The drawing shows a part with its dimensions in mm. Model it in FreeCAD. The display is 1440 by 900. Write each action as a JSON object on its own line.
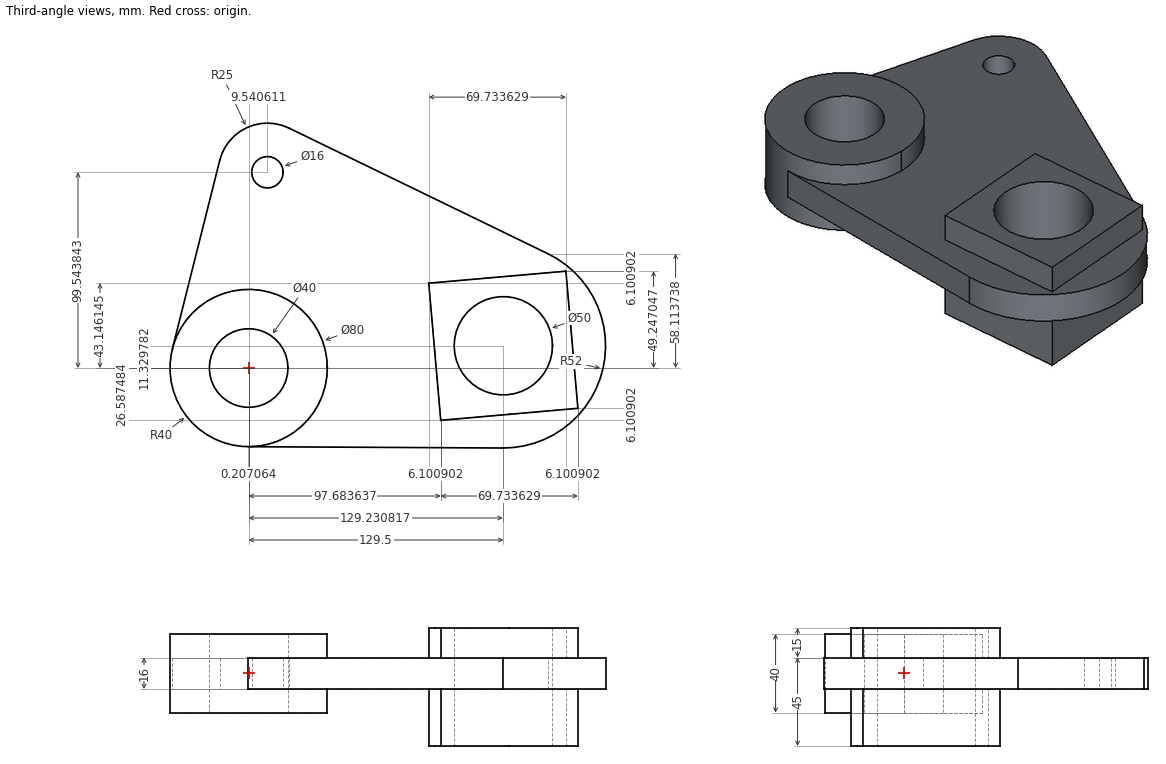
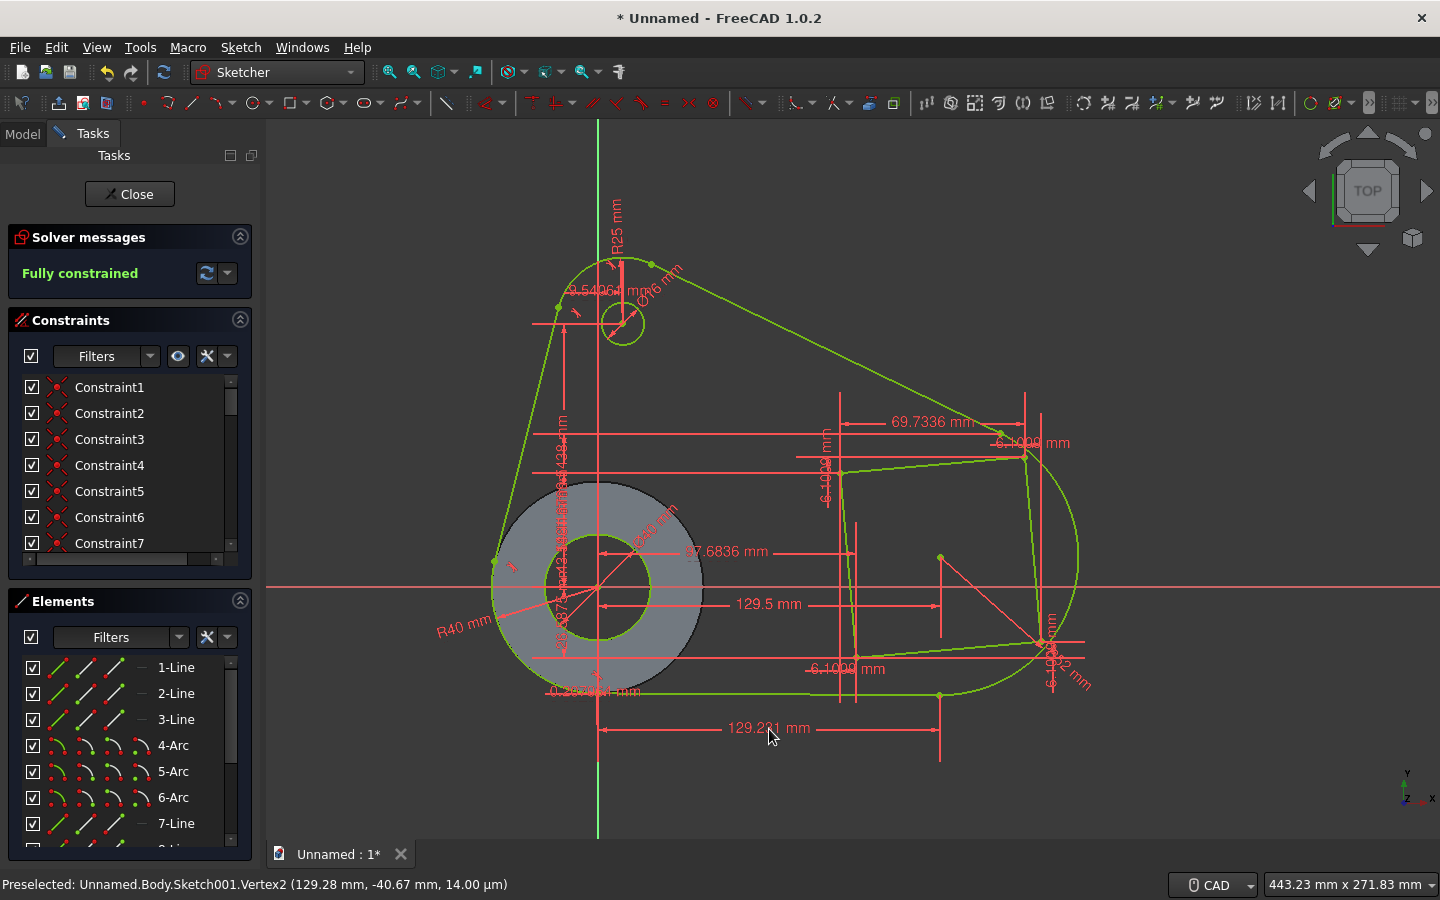
{"action": "left_click", "coordinate": [130, 194]}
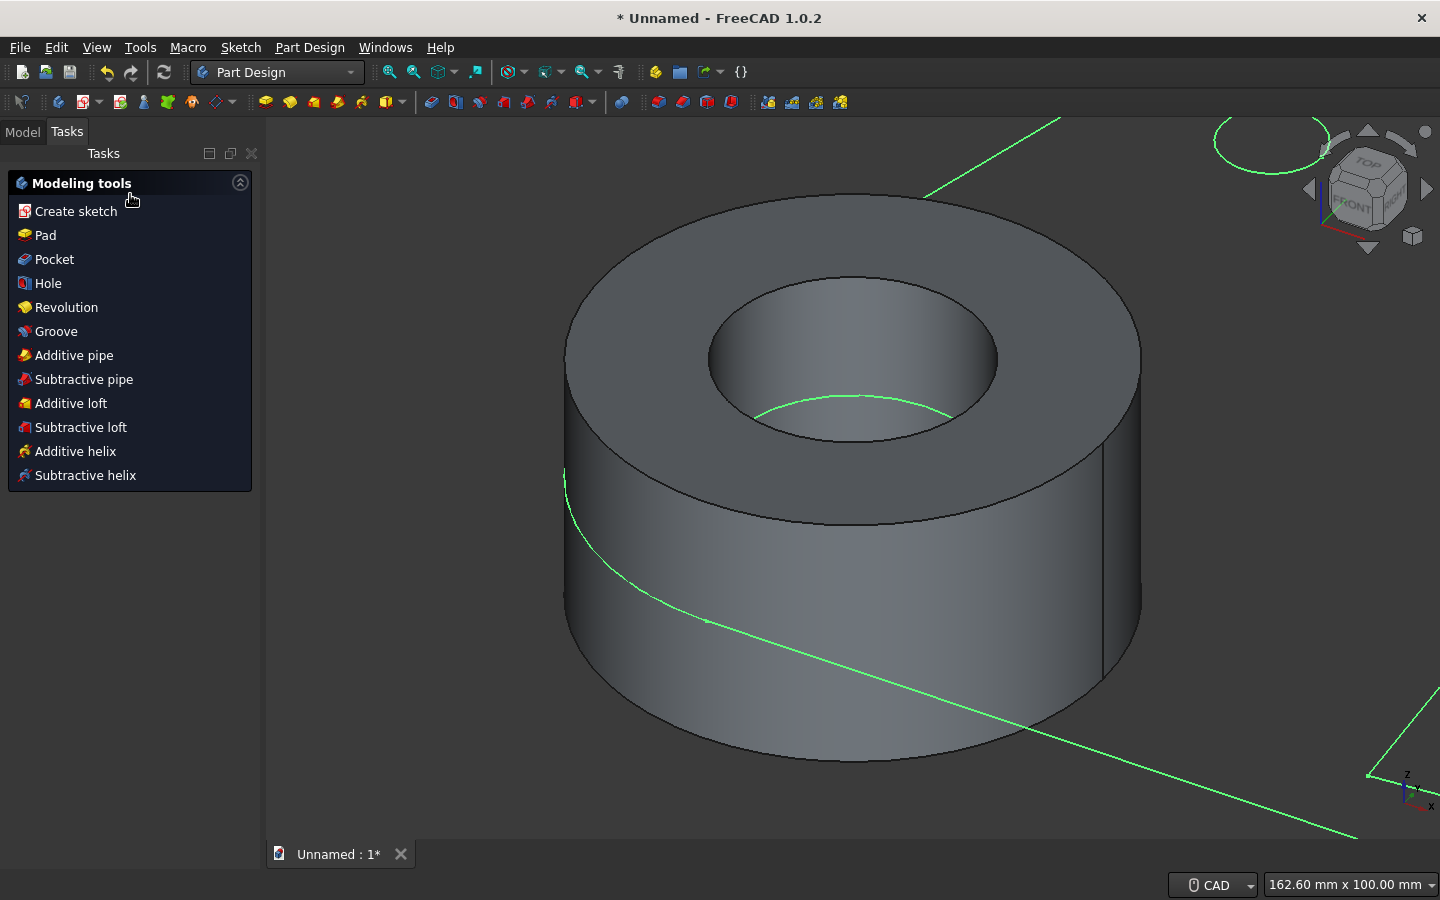
{"action": "left_click", "coordinate": [266, 102]}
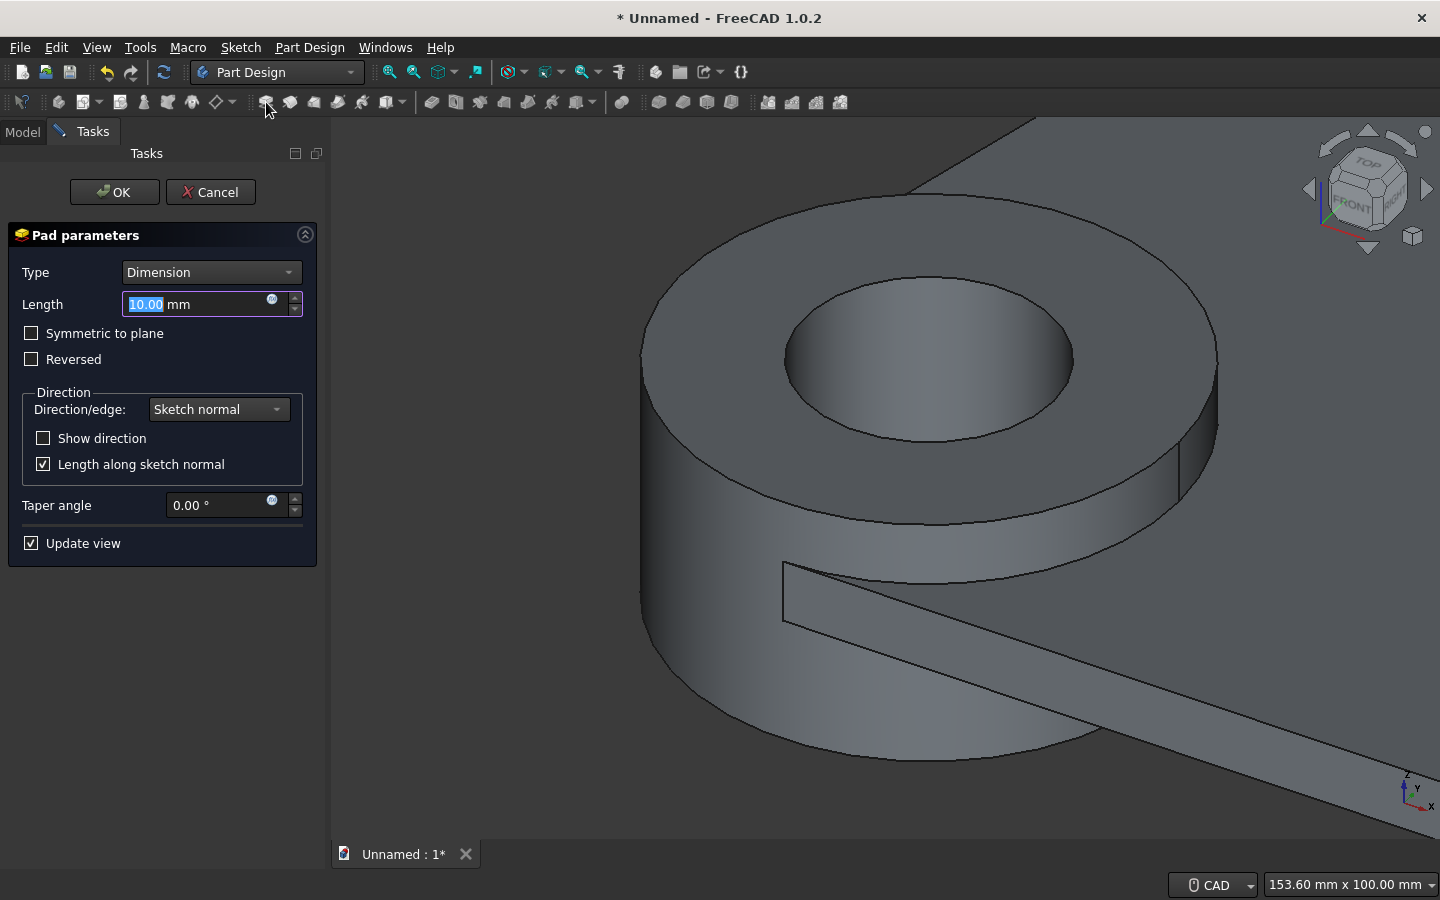
{"action": "type", "text": "16"}
{"action": "key", "text": "Tab"}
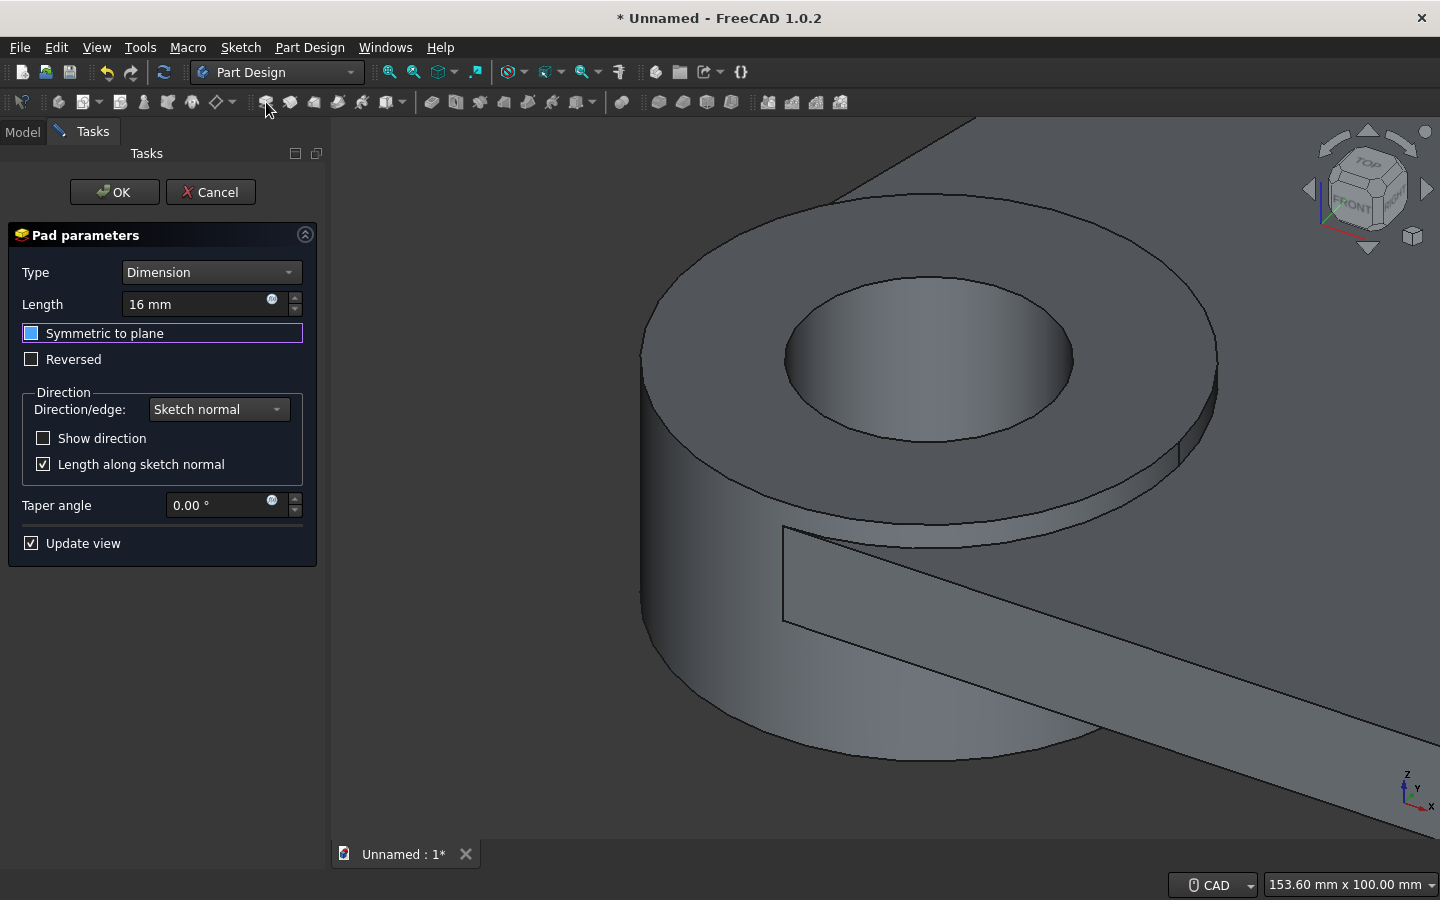
{"action": "left_click", "coordinate": [30, 333]}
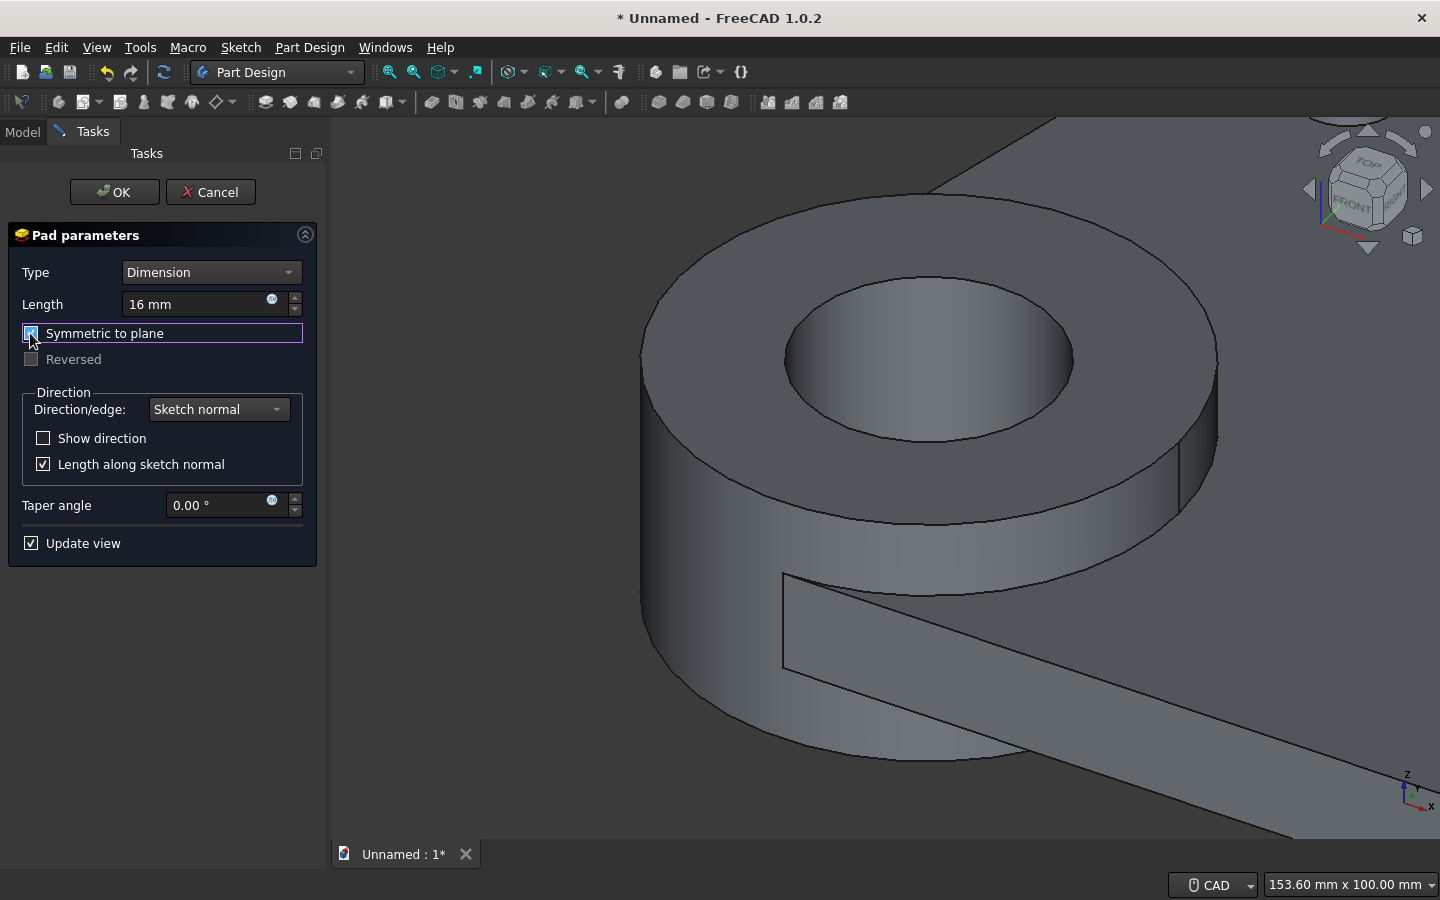
{"action": "left_click", "coordinate": [115, 192]}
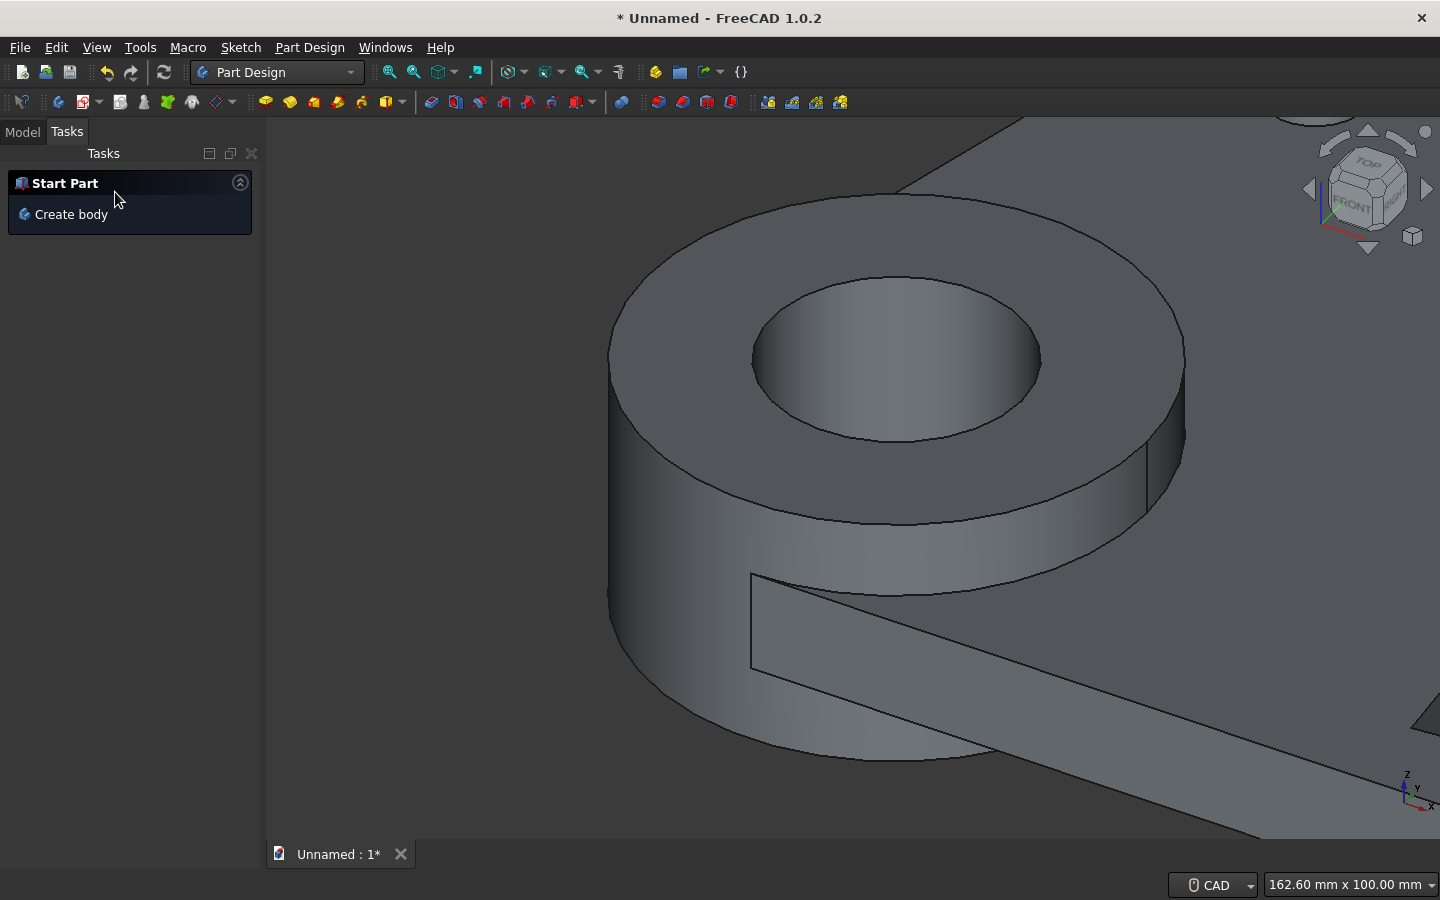
{"action": "left_click", "coordinate": [390, 72]}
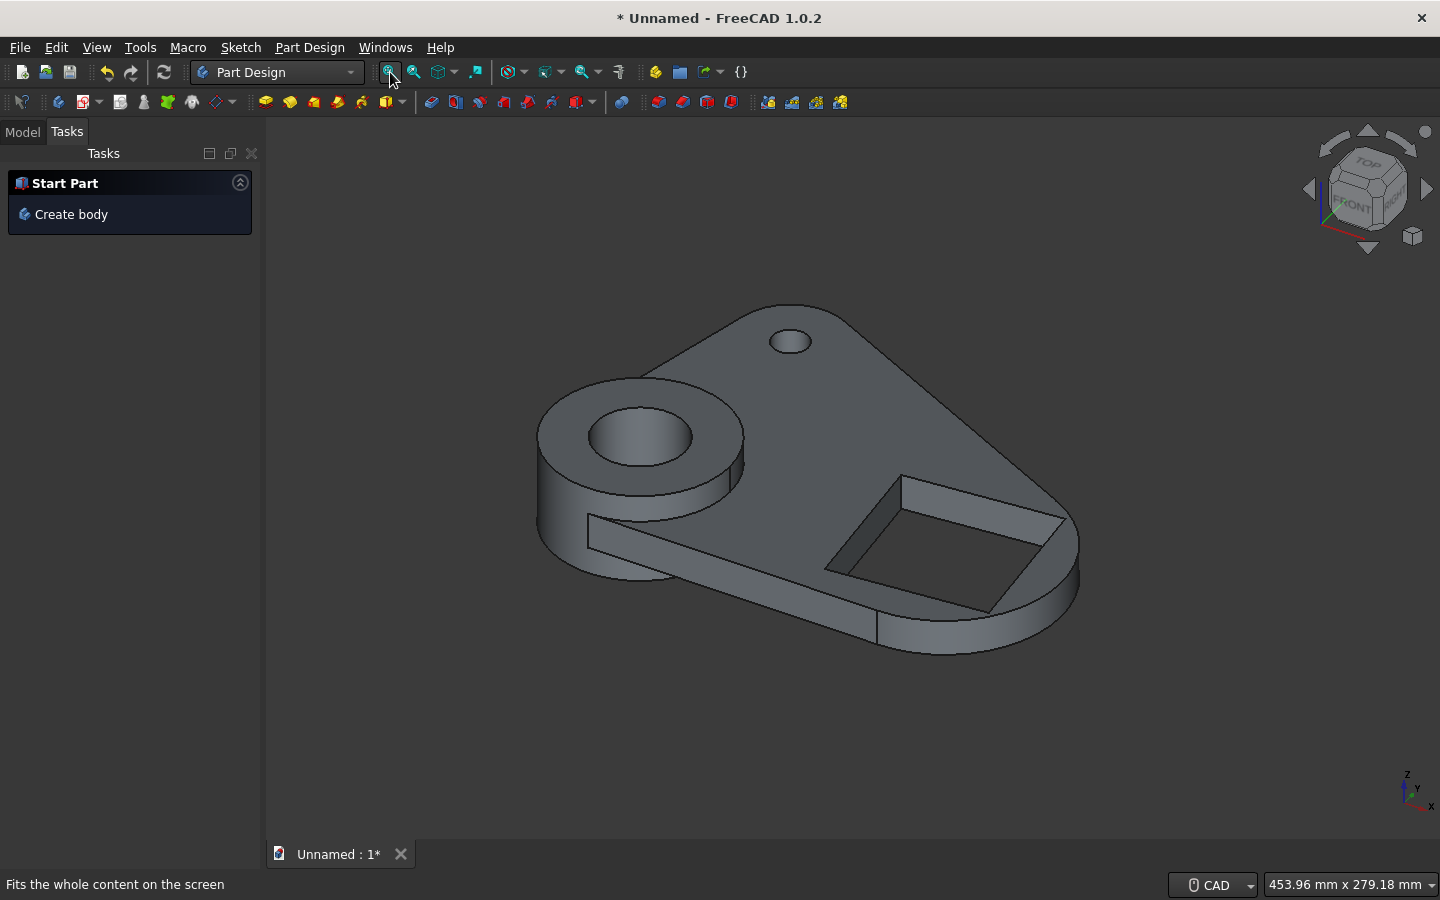
{"action": "left_click", "coordinate": [814, 407]}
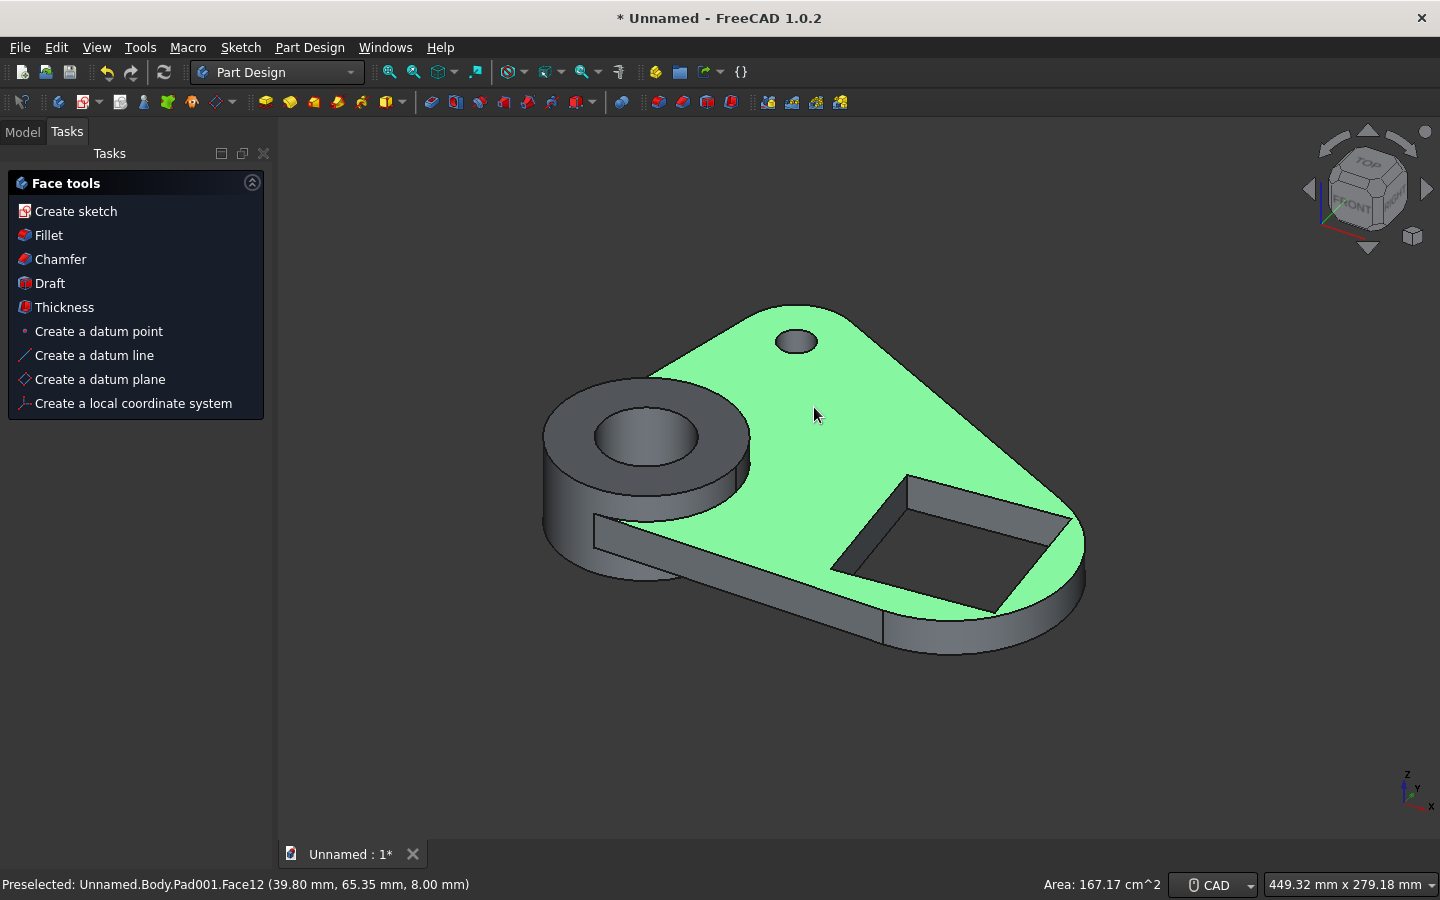
{"action": "left_click", "coordinate": [84, 102]}